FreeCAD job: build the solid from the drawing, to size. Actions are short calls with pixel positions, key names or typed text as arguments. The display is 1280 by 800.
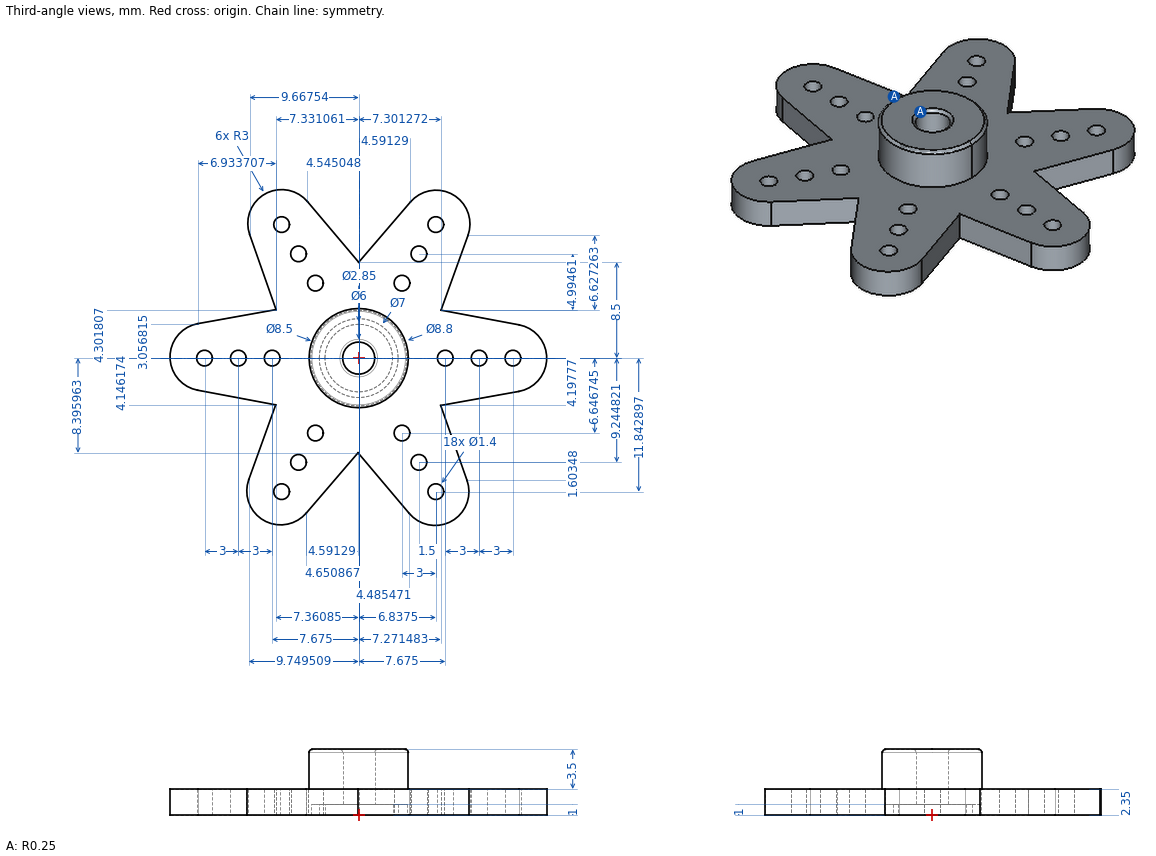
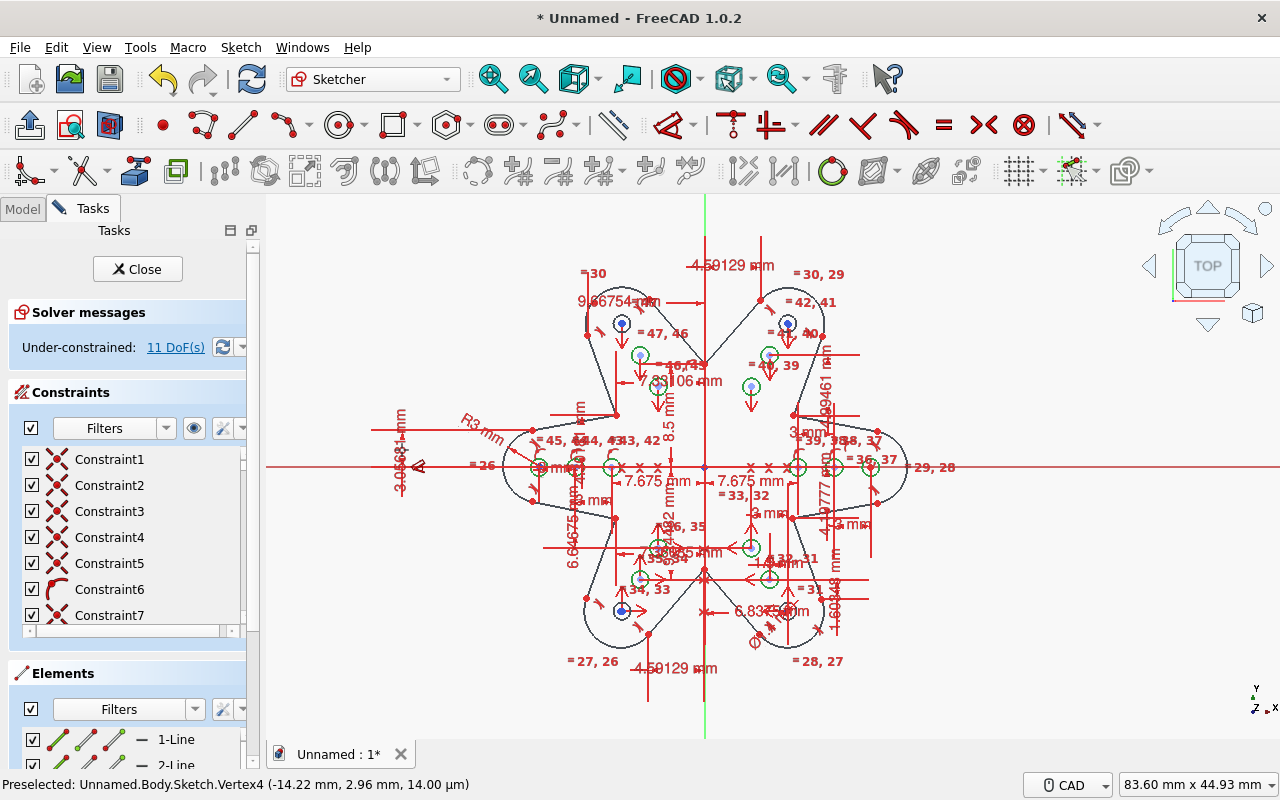
click(616, 519)
click(486, 493)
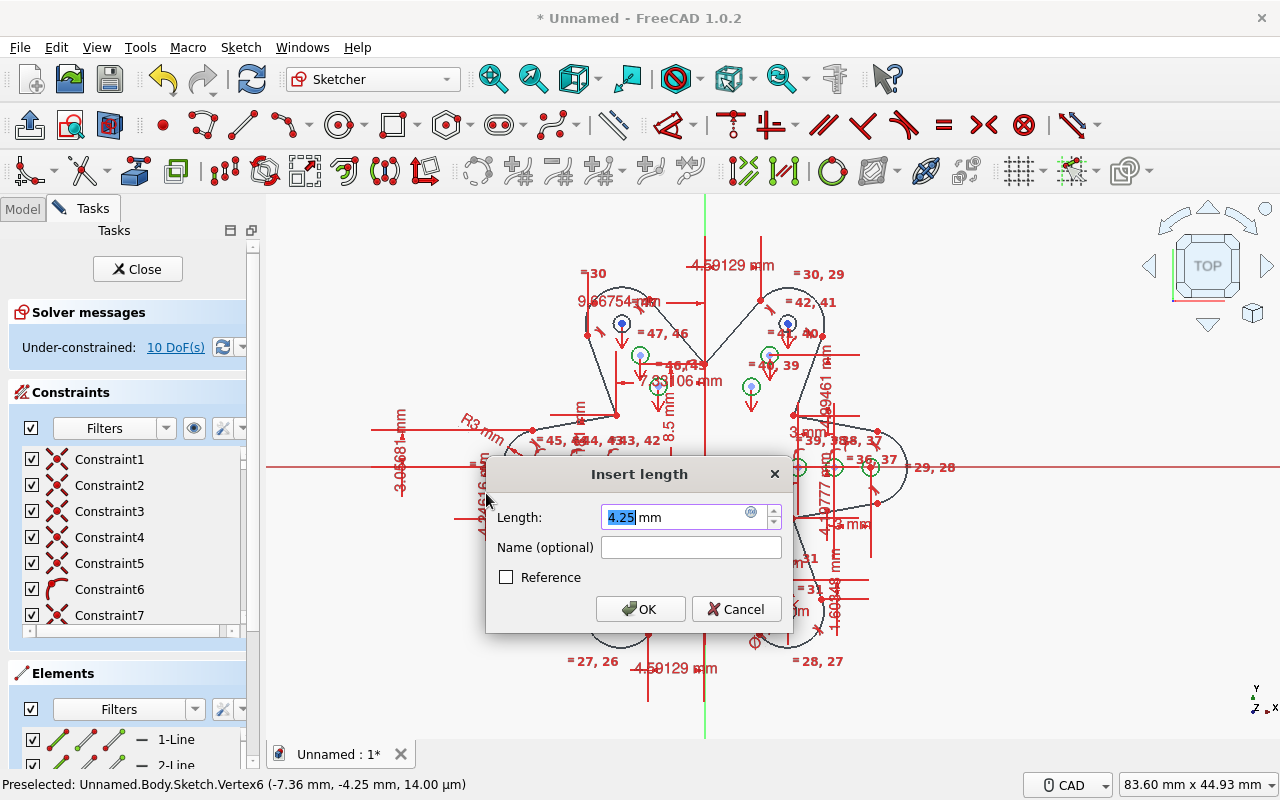
text(4.146174)
key(Return)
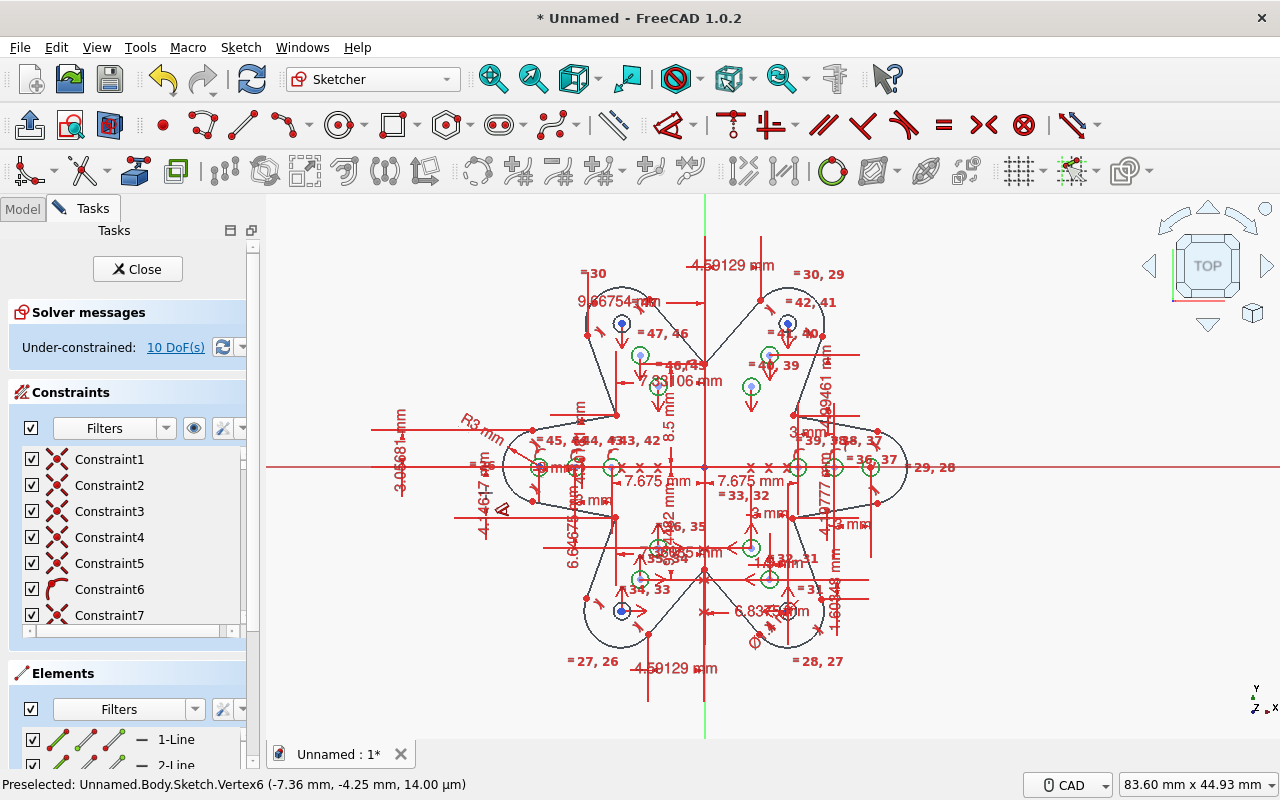
click(587, 599)
click(618, 633)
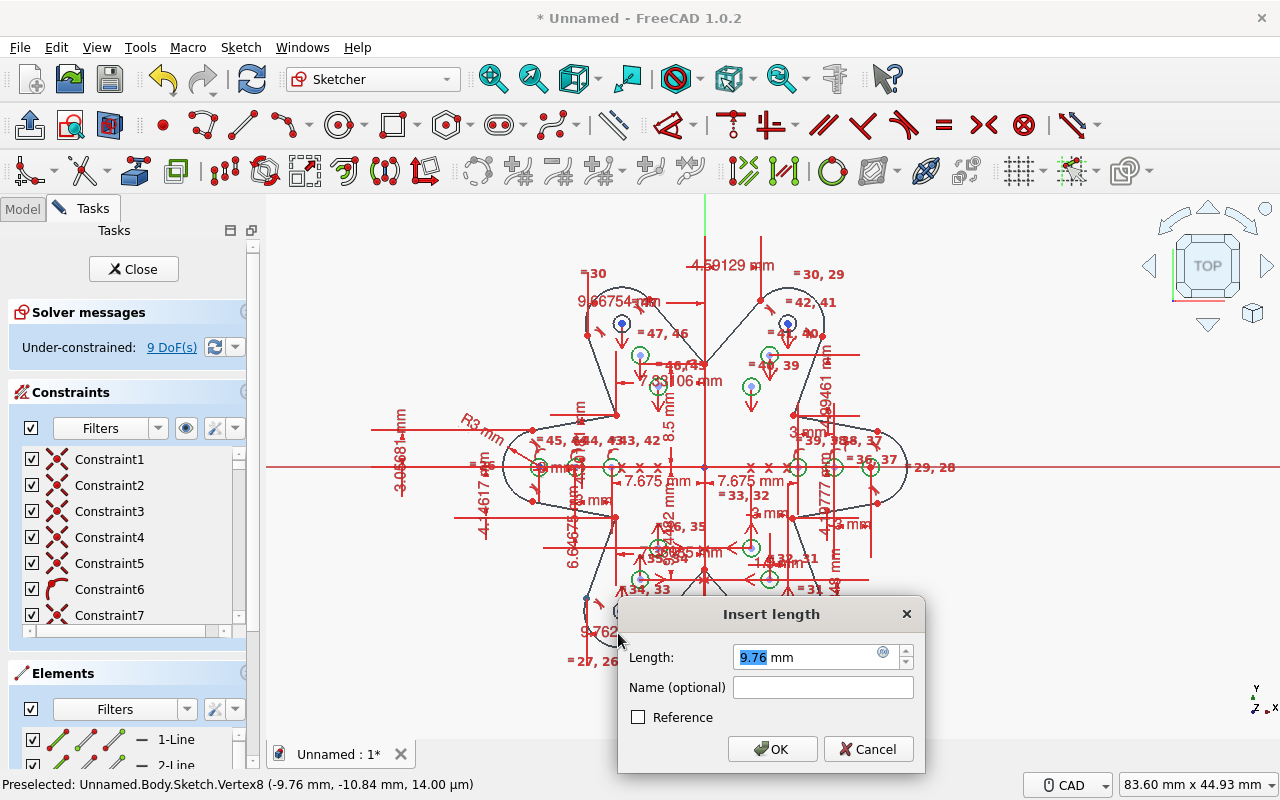
text(9.749509)
key(Return)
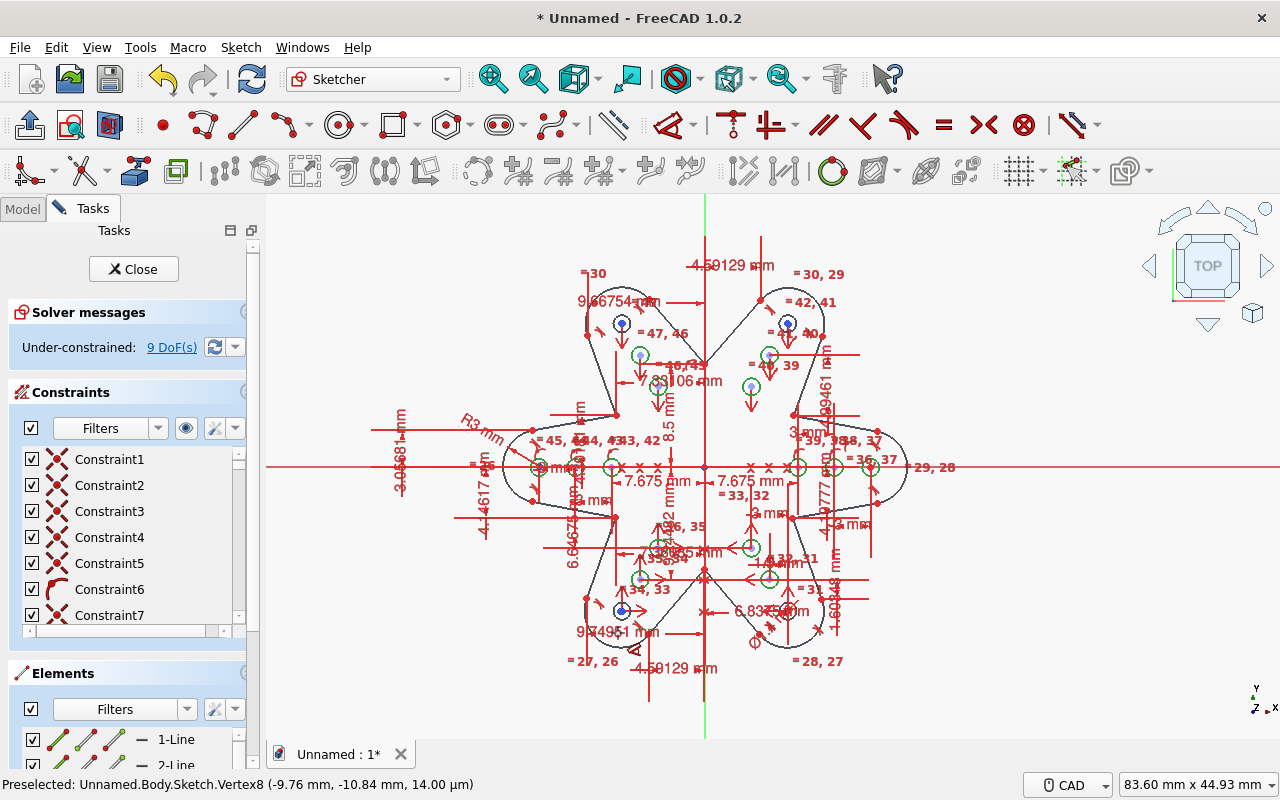
click(649, 635)
click(677, 693)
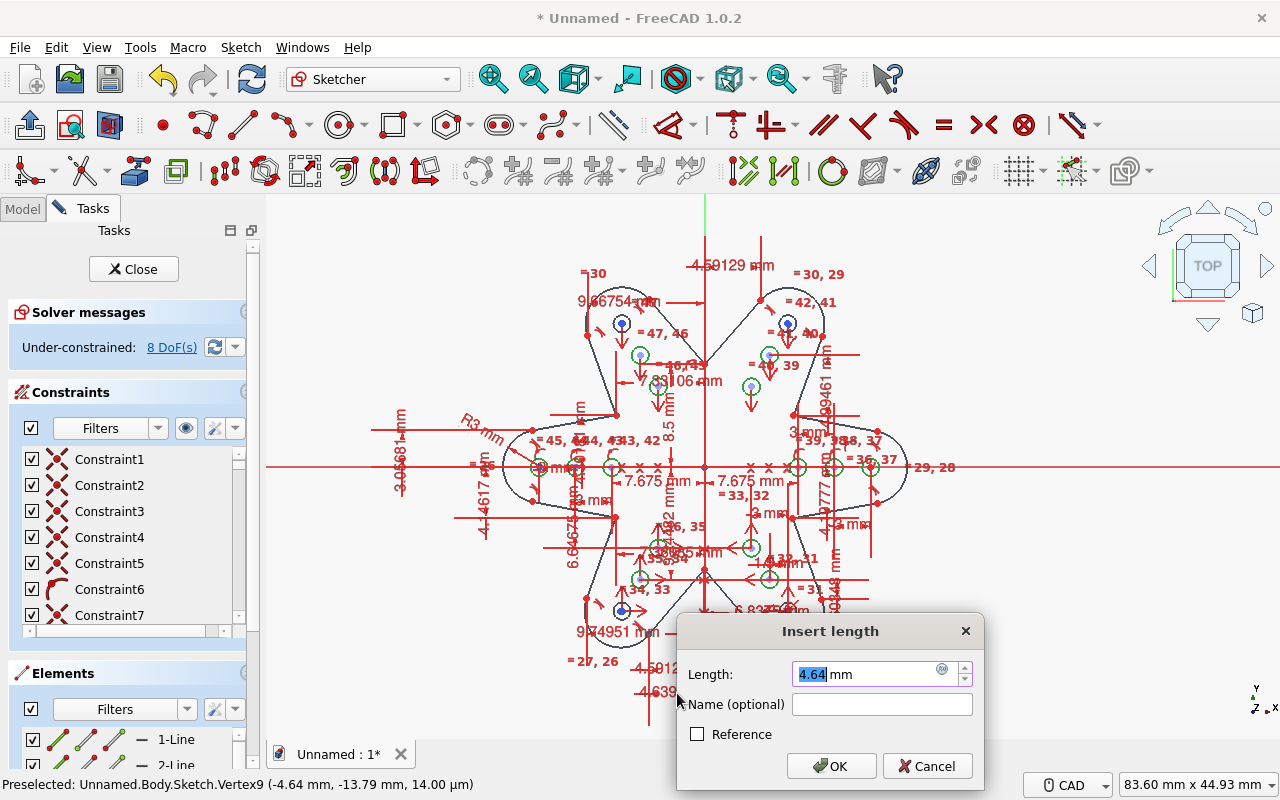
text(4.650867)
key(Return)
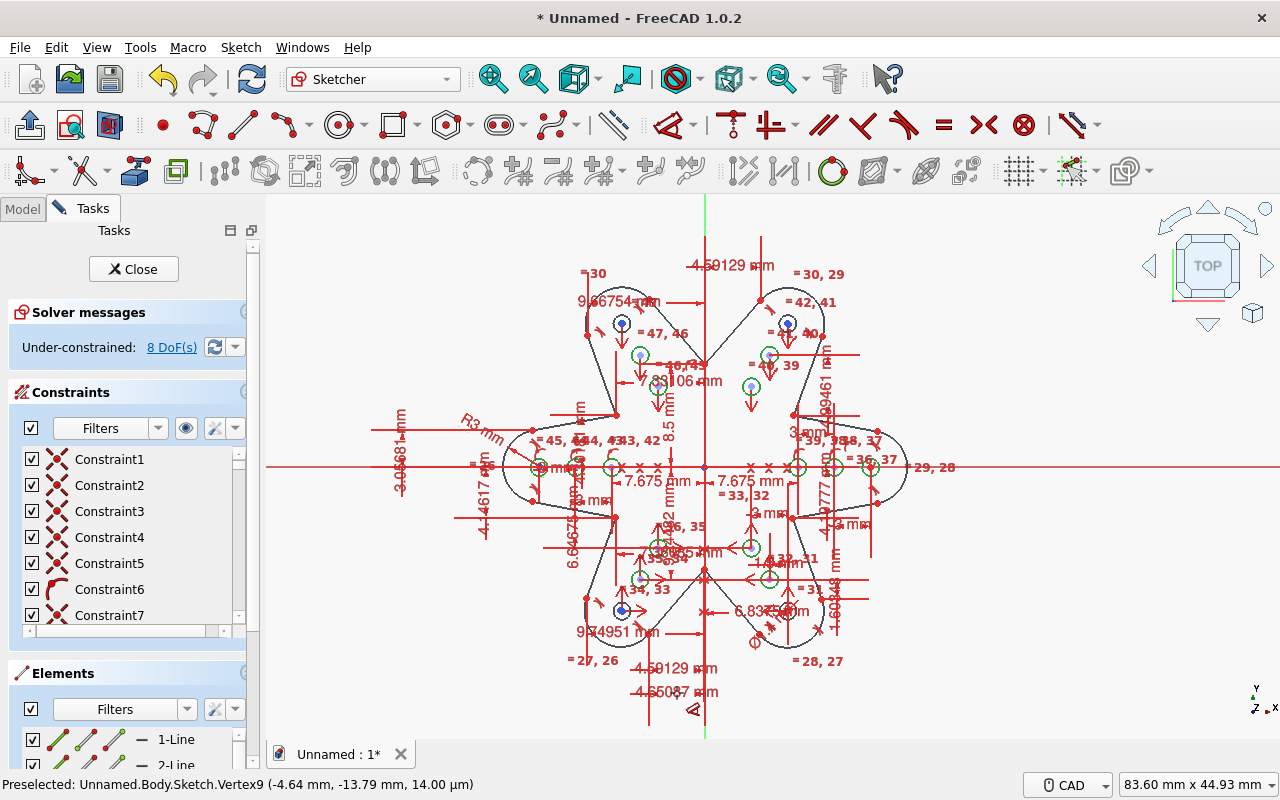
click(704, 569)
click(574, 554)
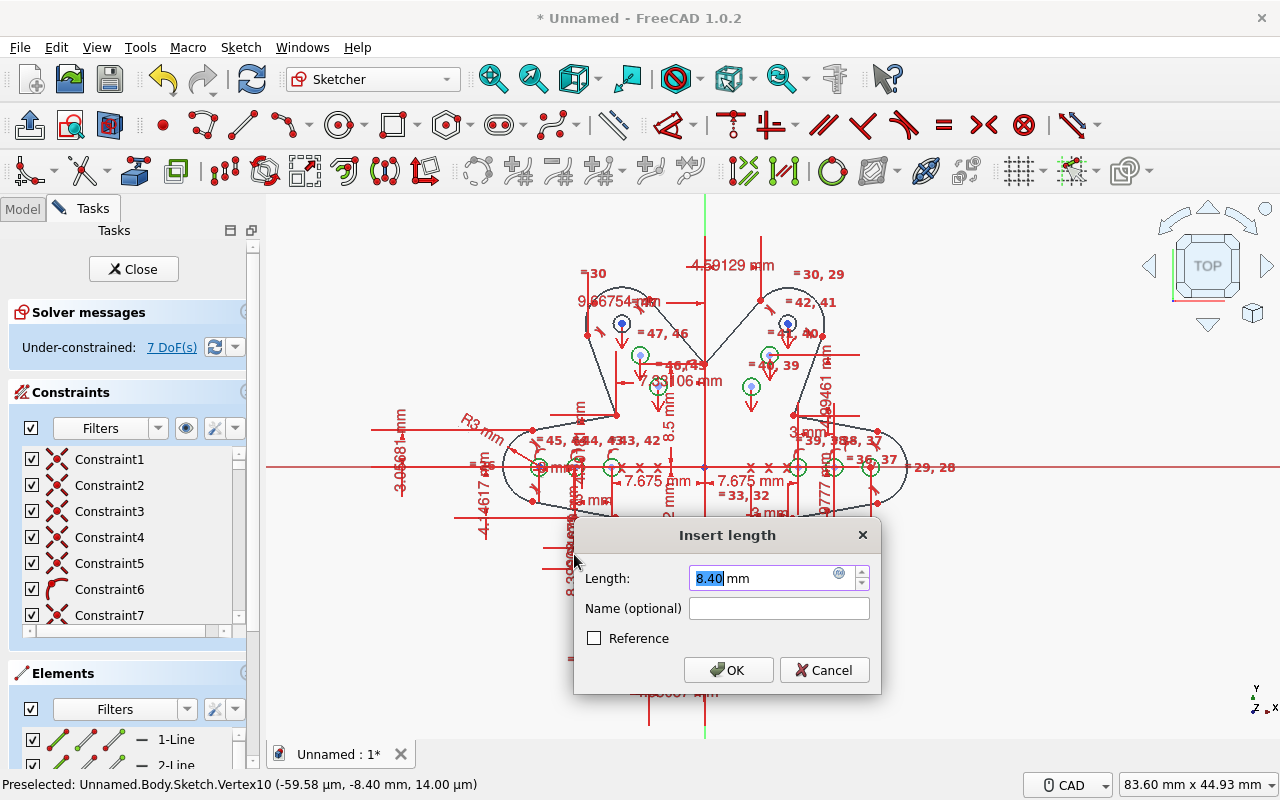
text(8.395963)
key(Return)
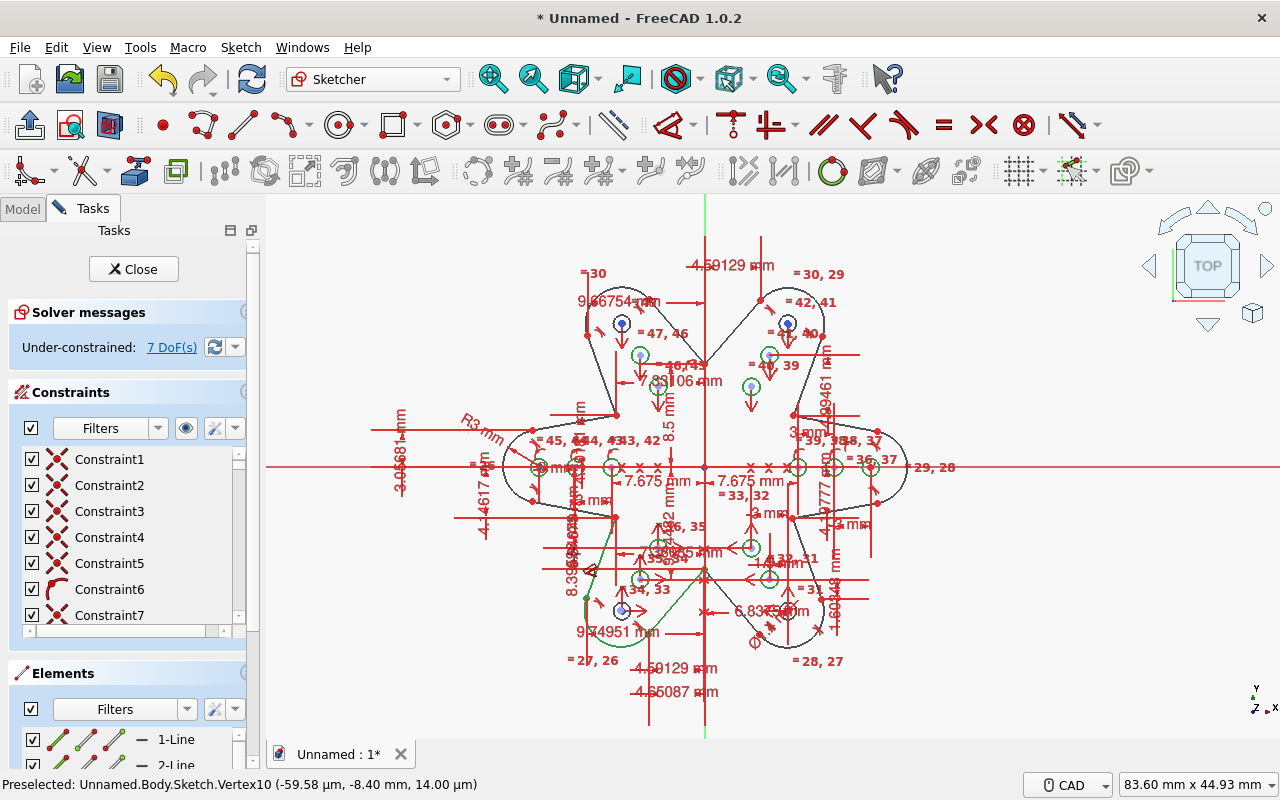
click(760, 635)
click(751, 669)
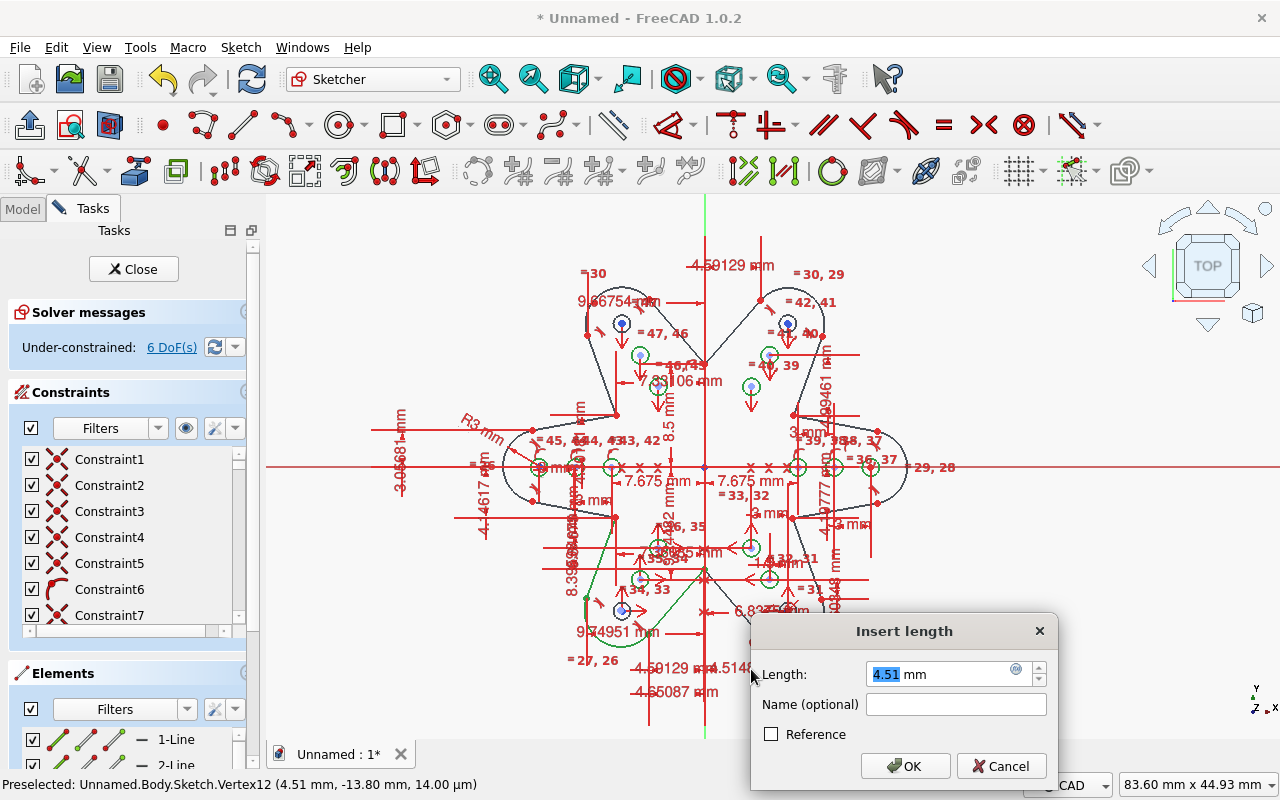
text(4.485471)
key(Return)